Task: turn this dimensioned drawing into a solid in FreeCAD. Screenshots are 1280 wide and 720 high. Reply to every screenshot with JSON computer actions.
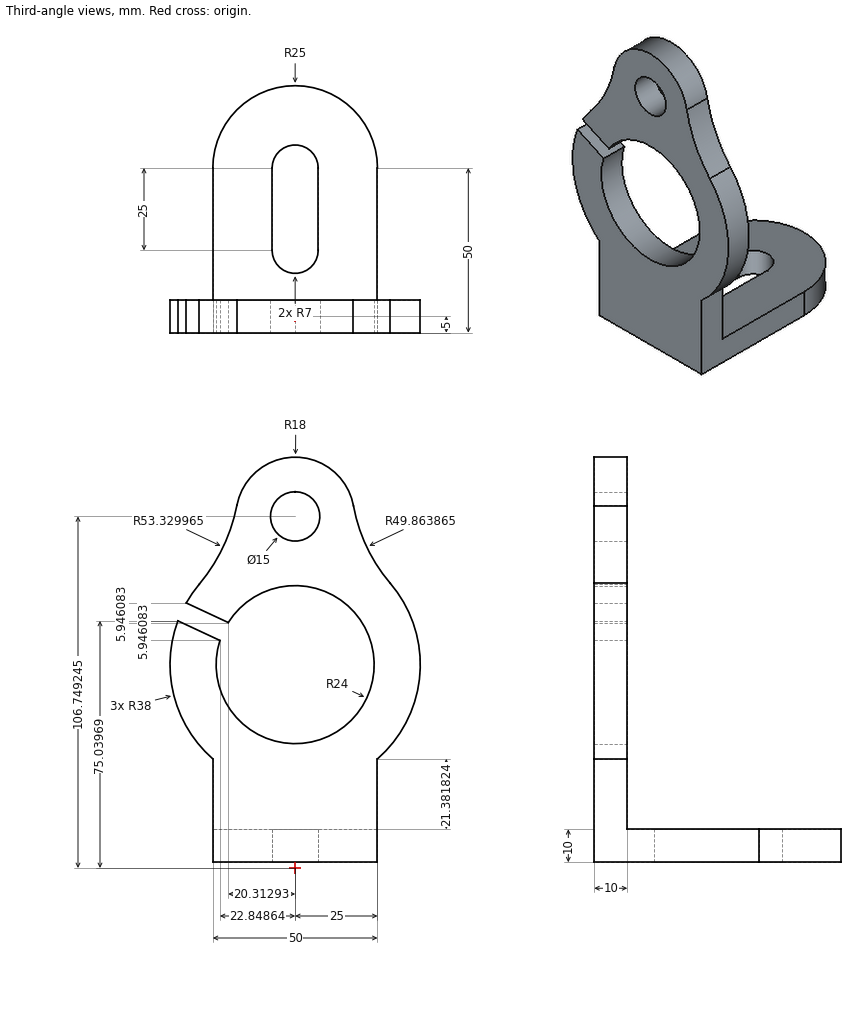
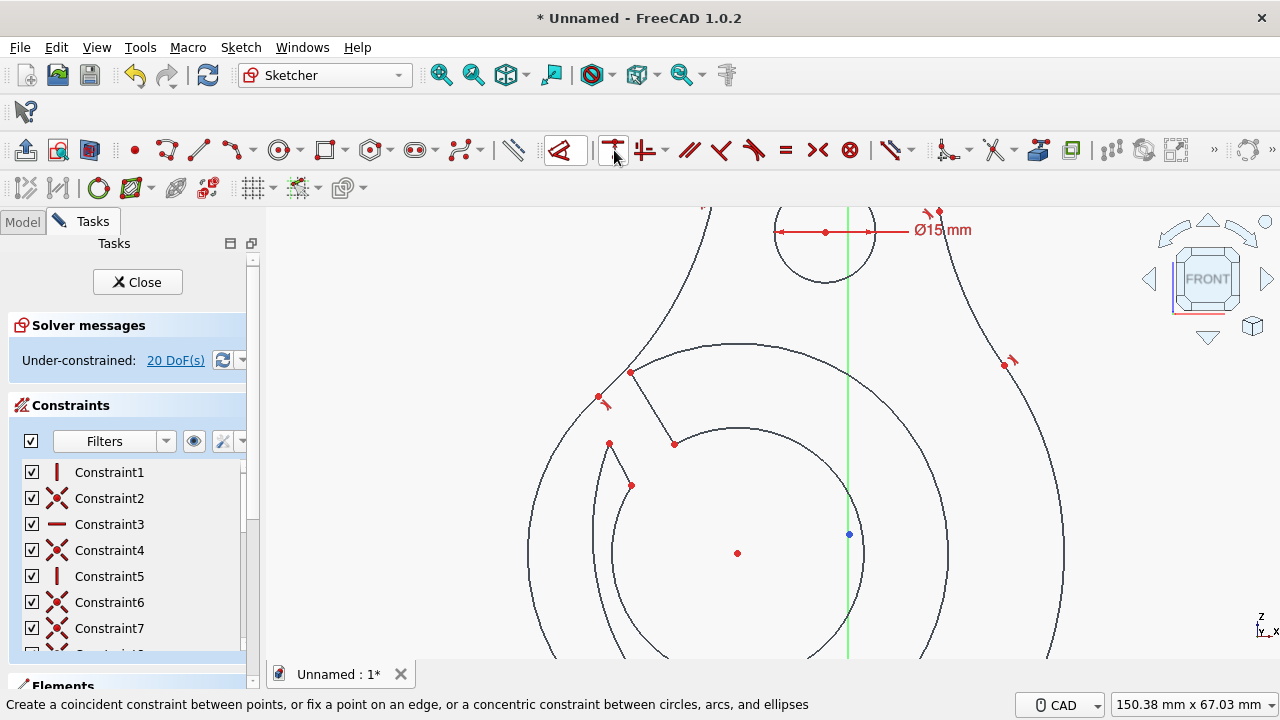
{"action": "left_click", "coordinate": [633, 624]}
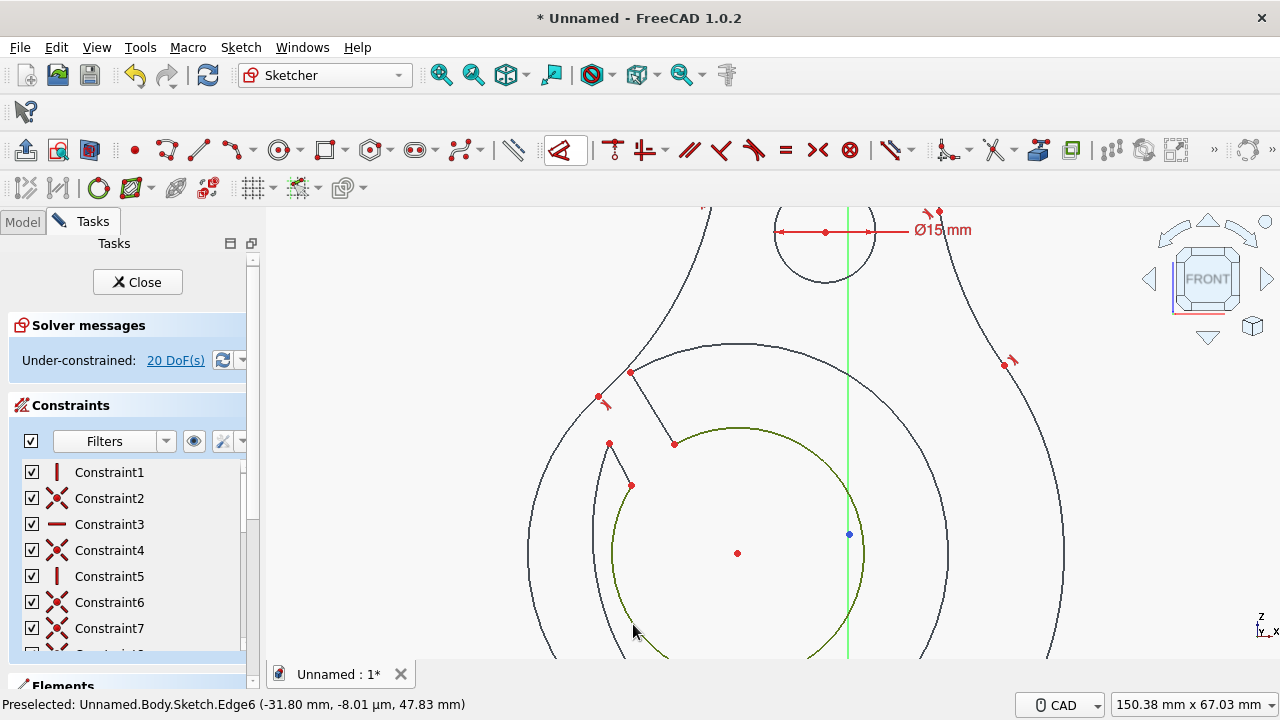
{"action": "left_click", "coordinate": [593, 535]}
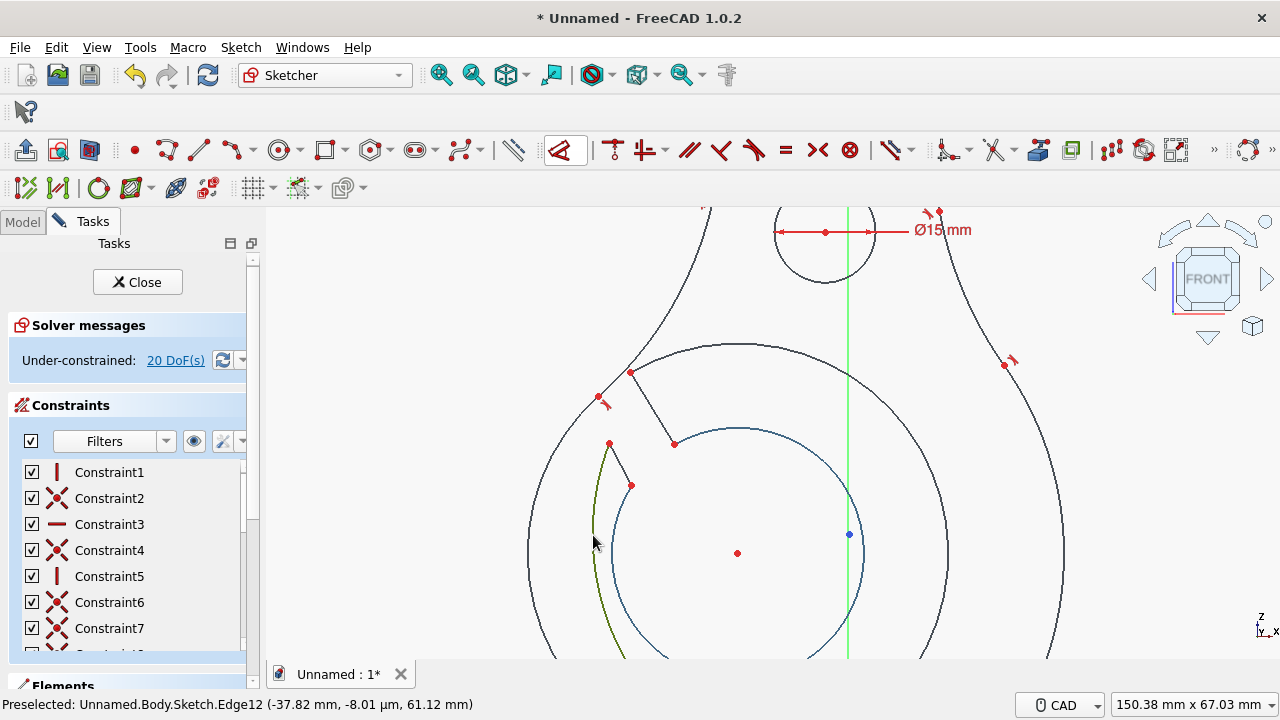
{"action": "left_click", "coordinate": [614, 150]}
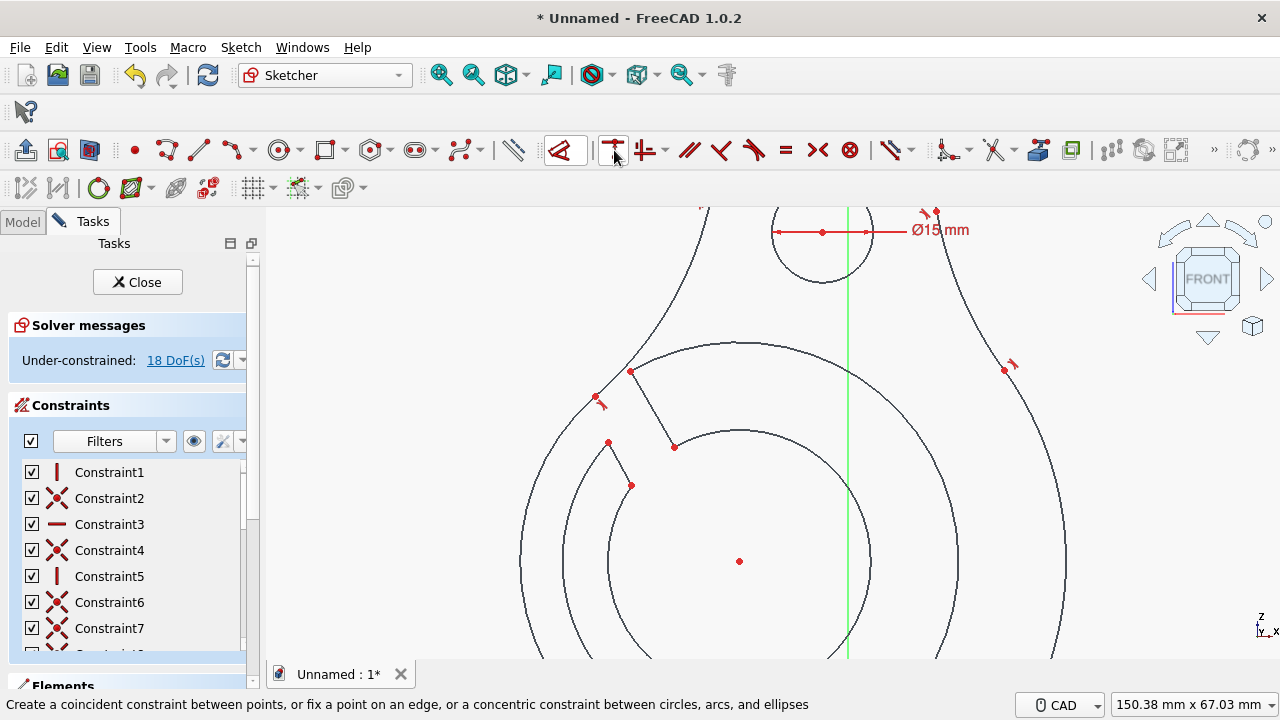
{"action": "left_click", "coordinate": [951, 504]}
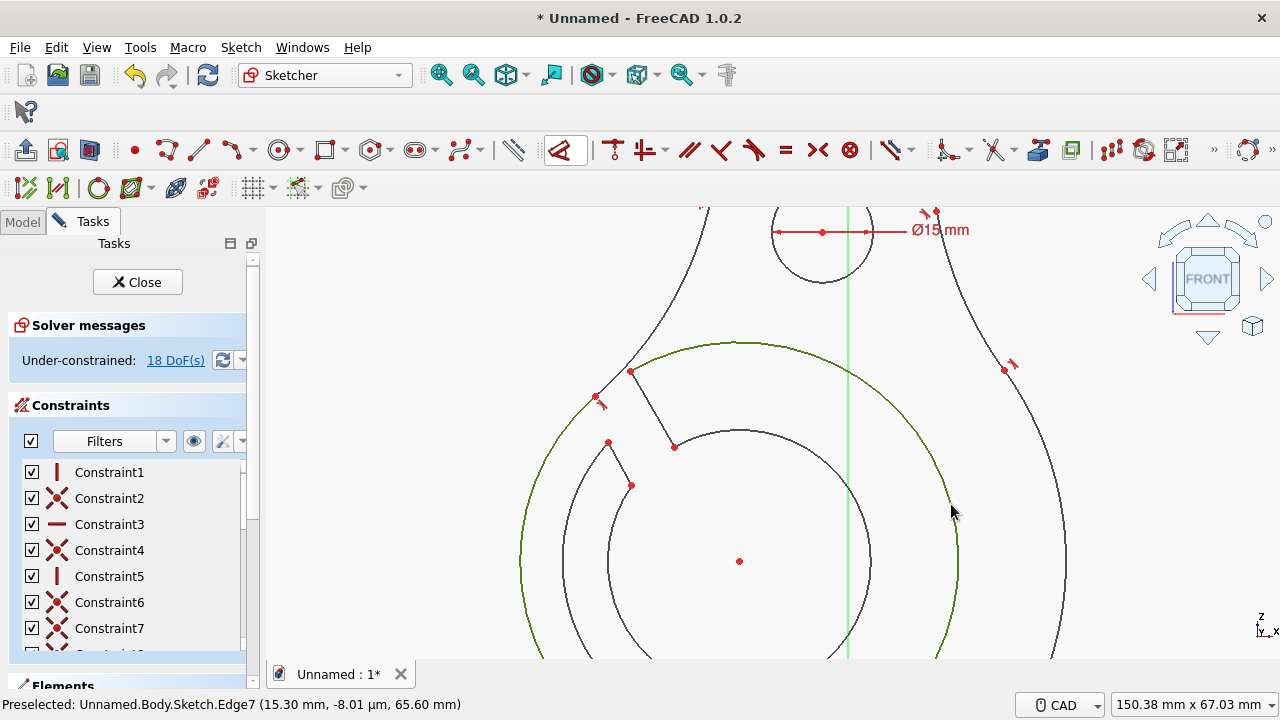
{"action": "left_click", "coordinate": [1061, 621]}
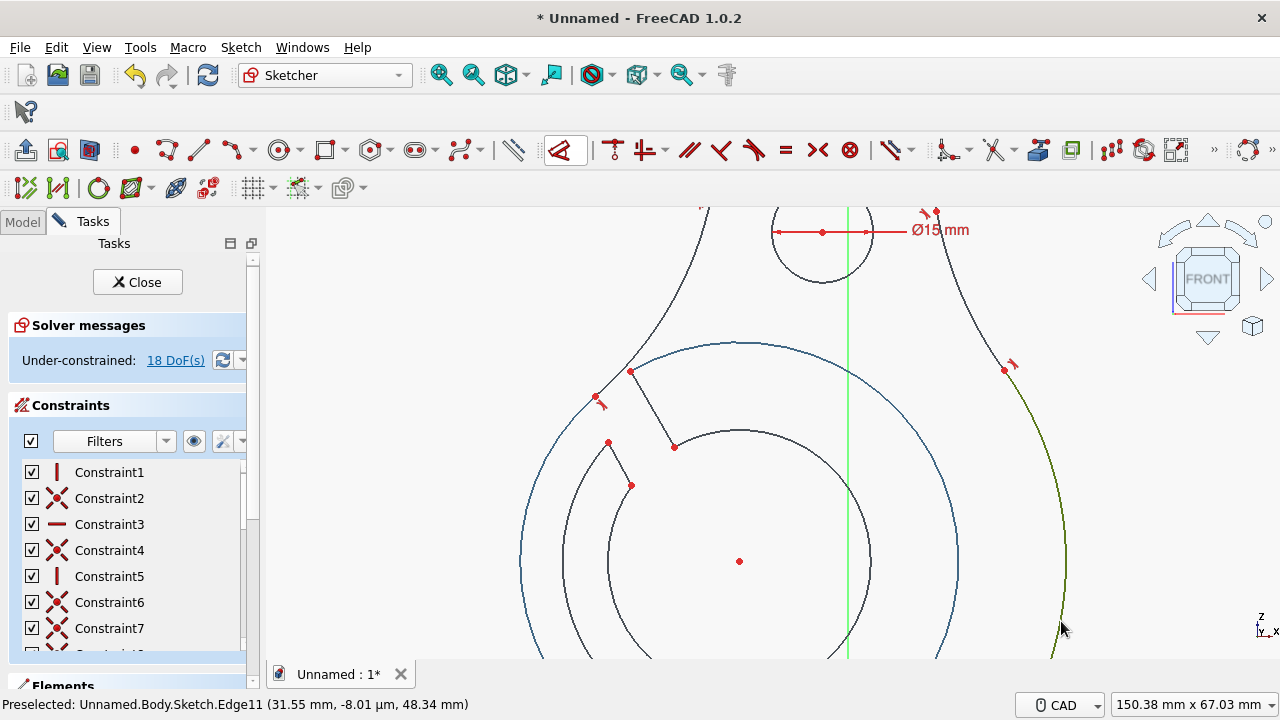
{"action": "left_click", "coordinate": [565, 535]}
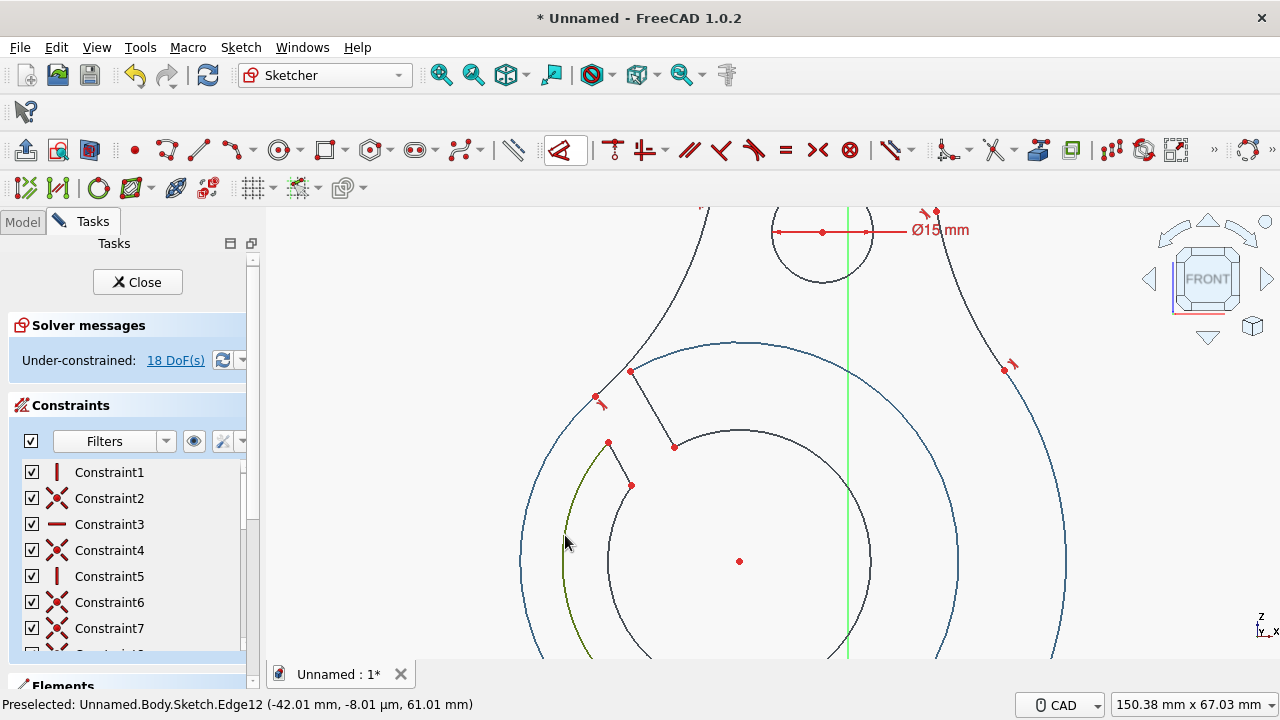
{"action": "left_click", "coordinate": [786, 150]}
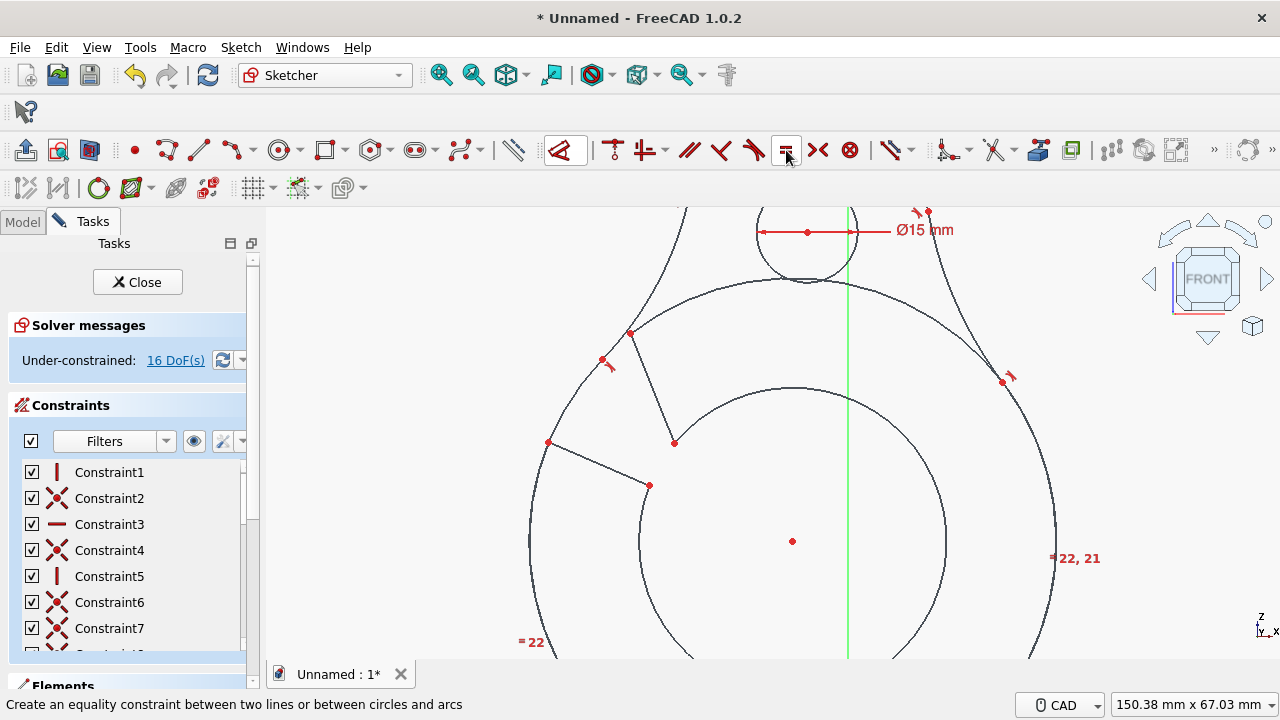
{"action": "left_click", "coordinate": [793, 542]}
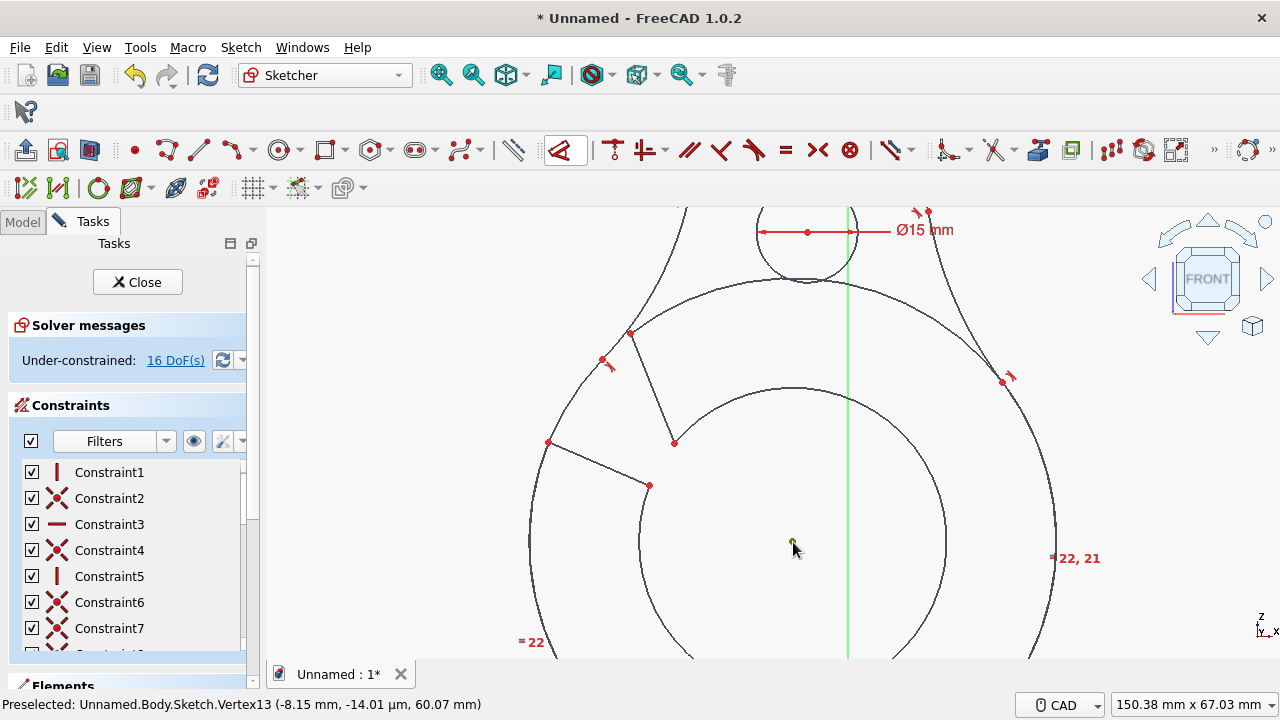
{"action": "left_click", "coordinate": [848, 603]}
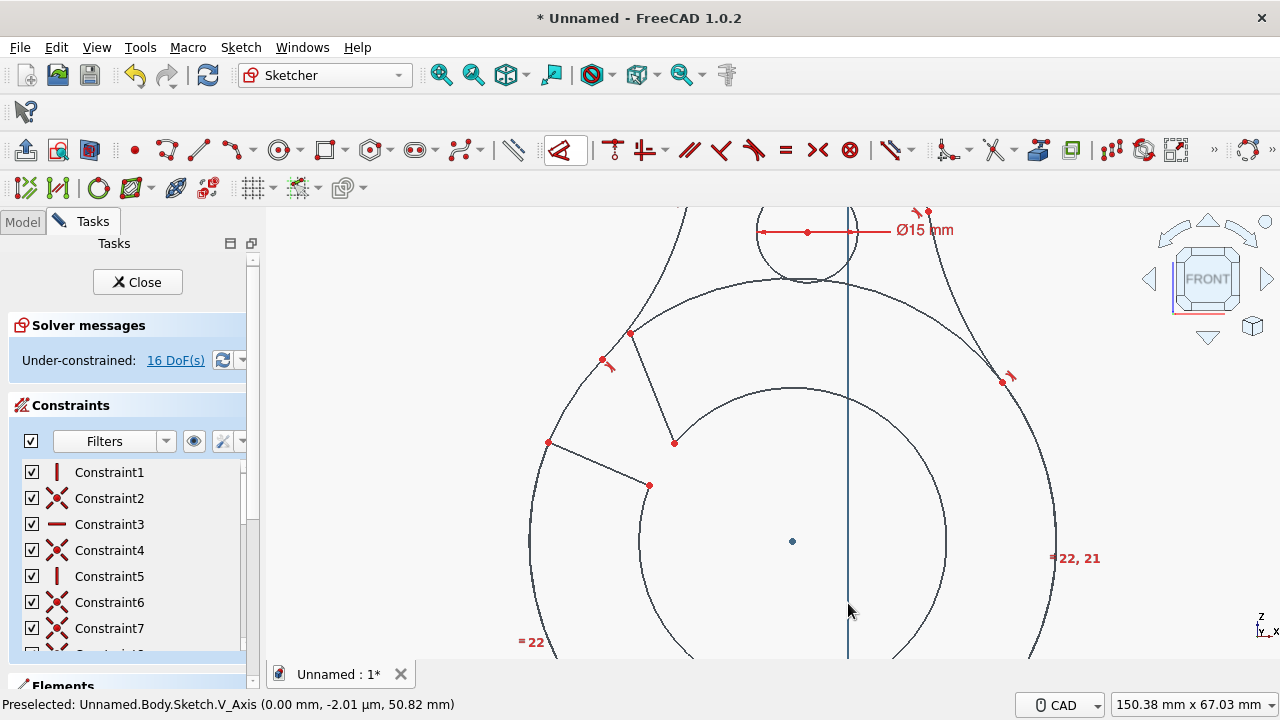
{"action": "left_click", "coordinate": [614, 150]}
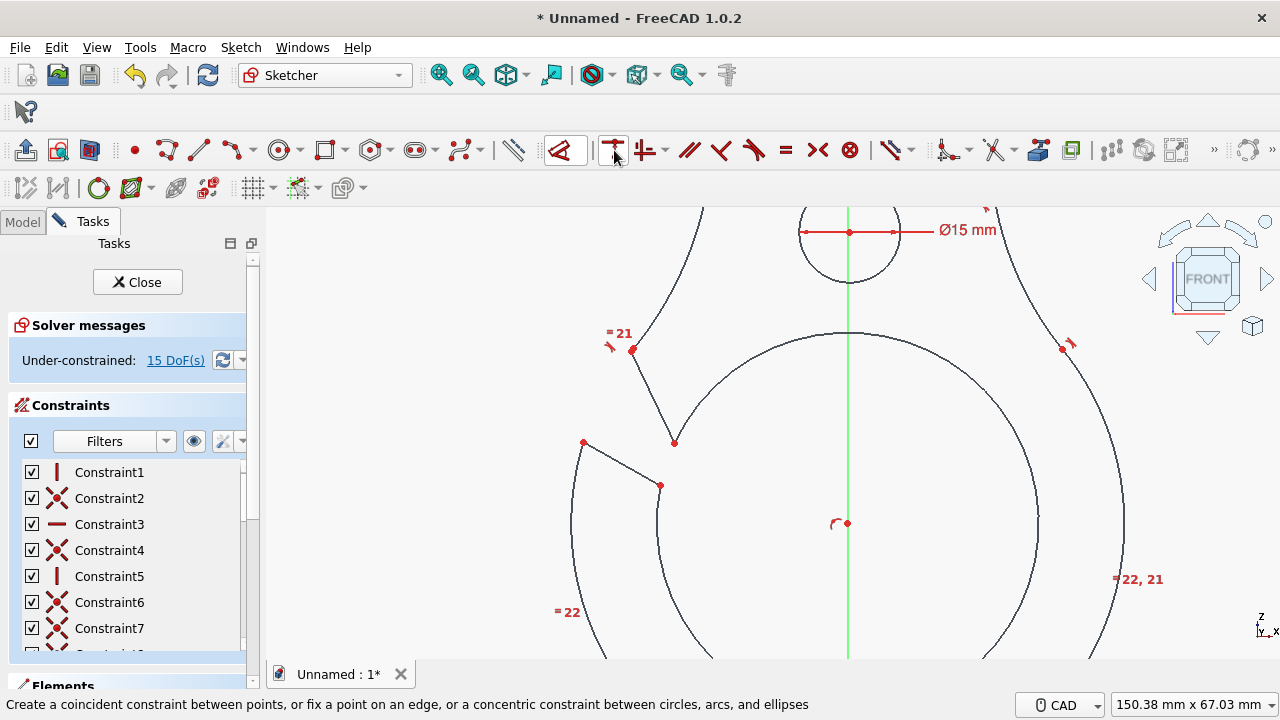
{"action": "scroll", "coordinate": [641, 393], "scroll_direction": "down", "scroll_amount": 6}